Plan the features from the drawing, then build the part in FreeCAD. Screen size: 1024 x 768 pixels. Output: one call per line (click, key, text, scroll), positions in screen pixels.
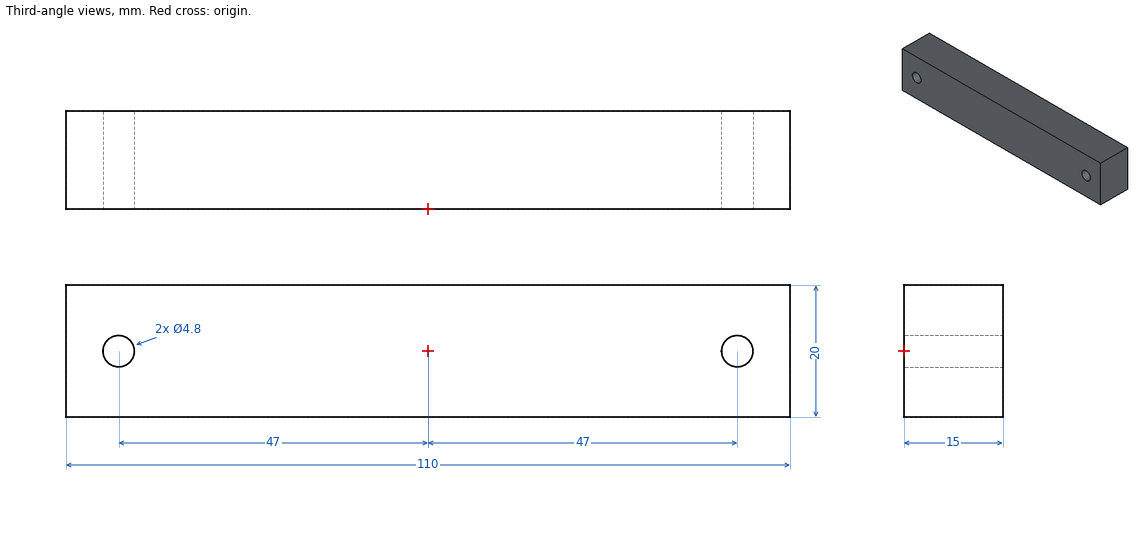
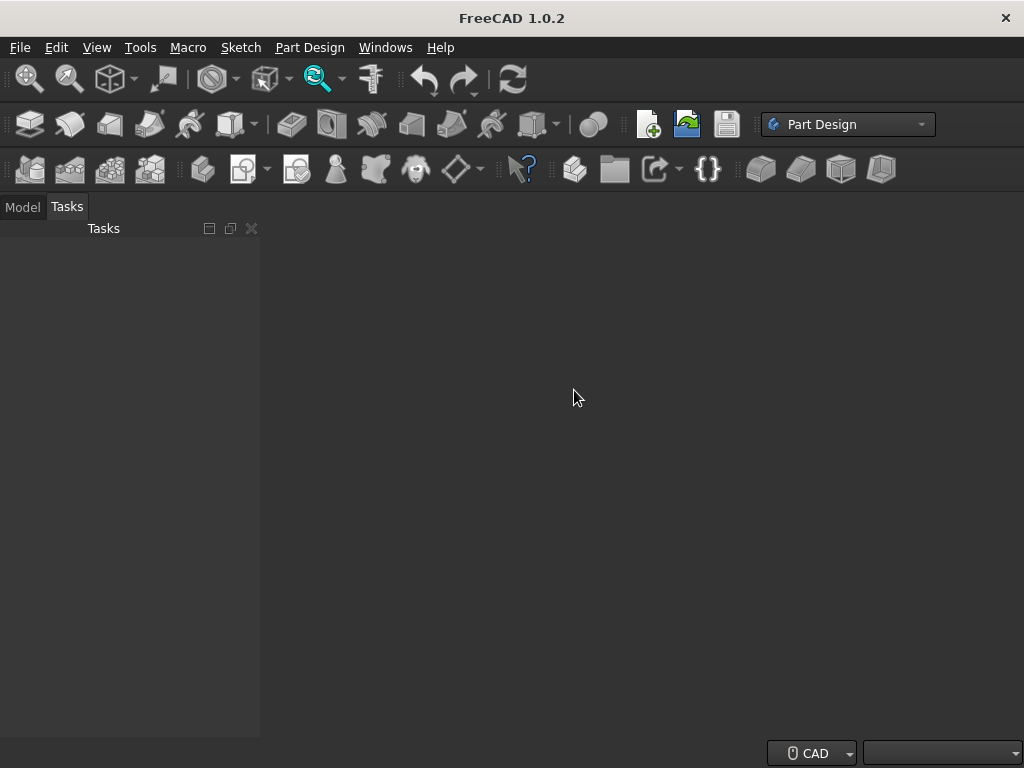
key(ctrl+n)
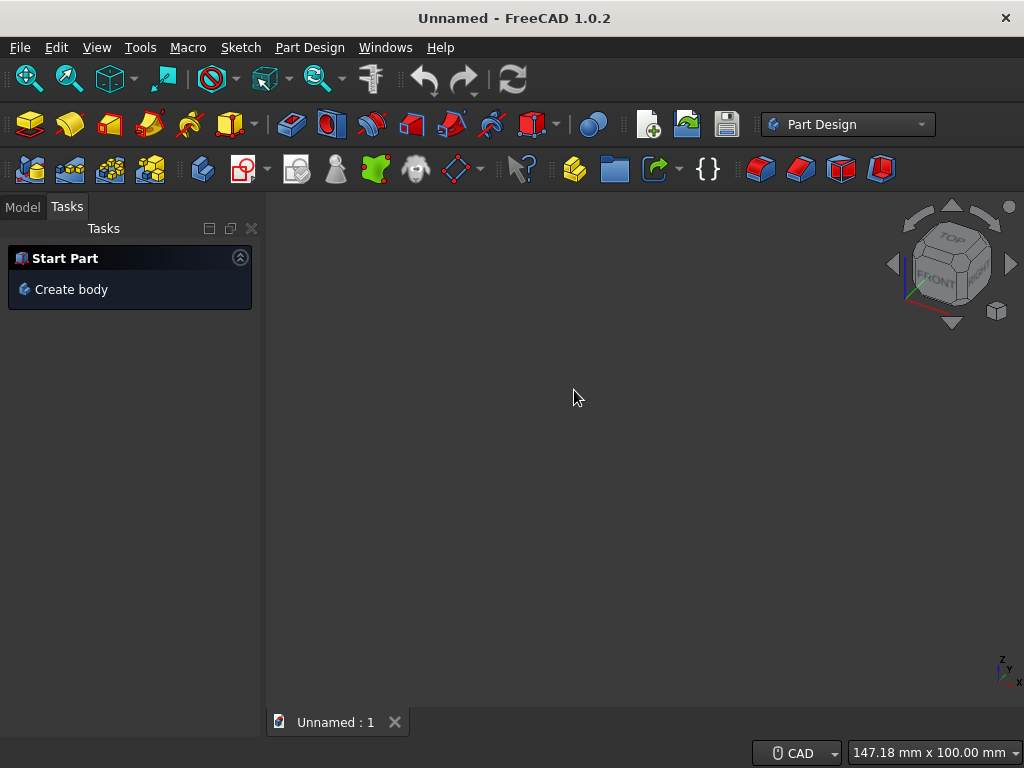
click(244, 170)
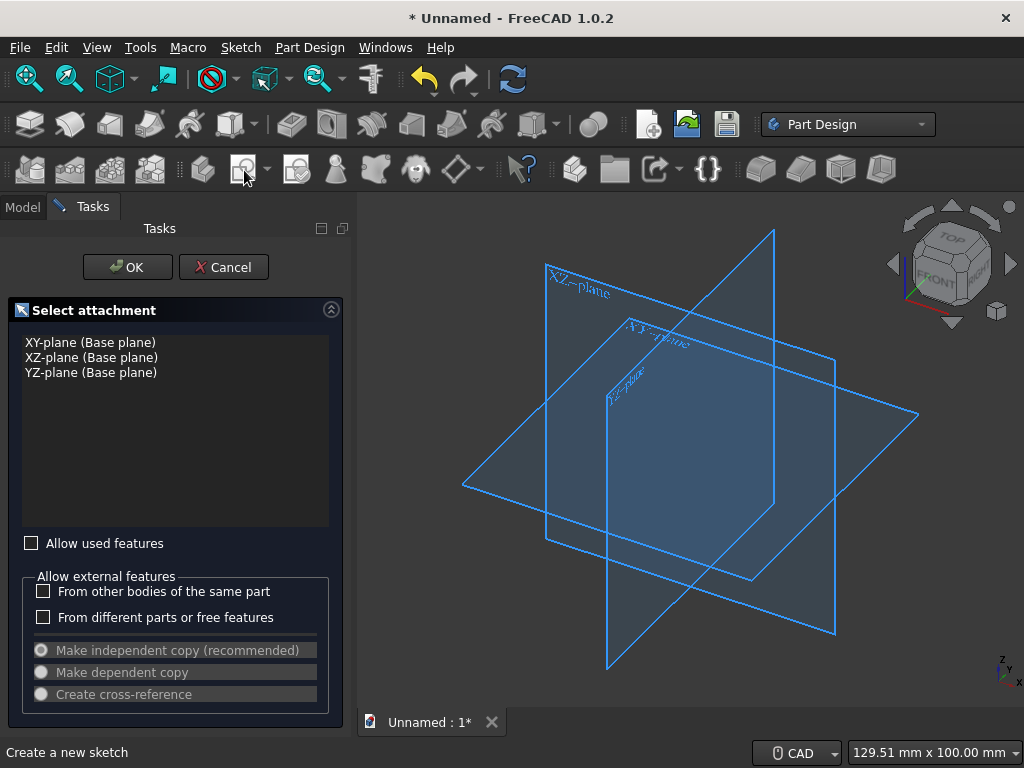
click(82, 358)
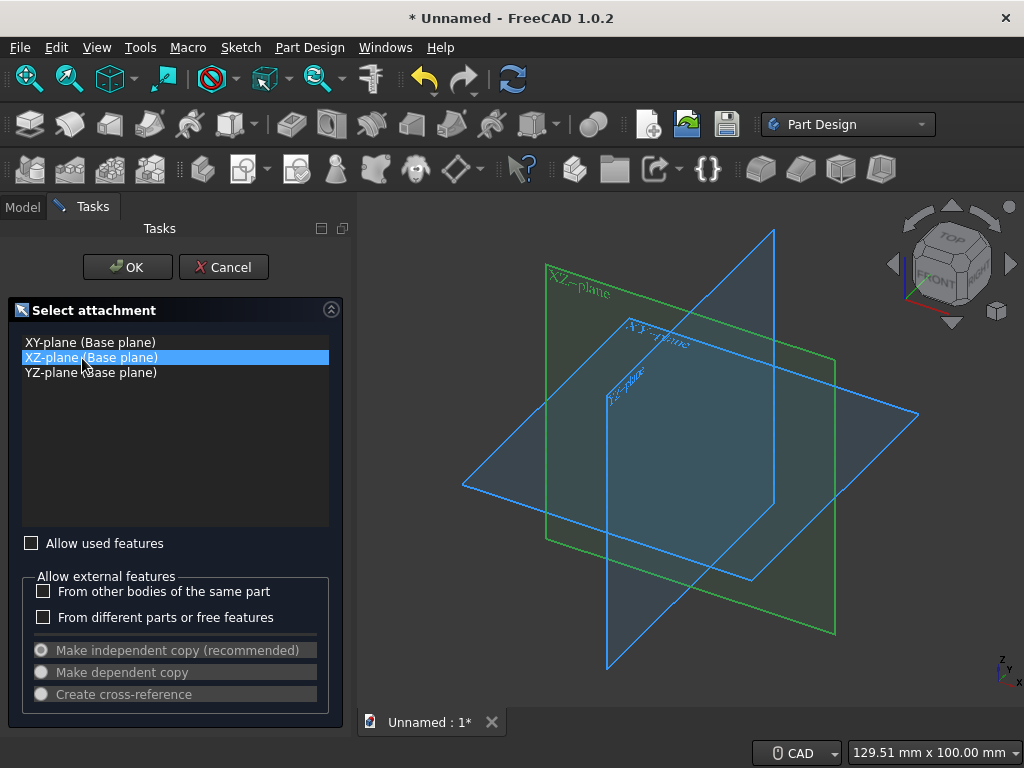
click(128, 267)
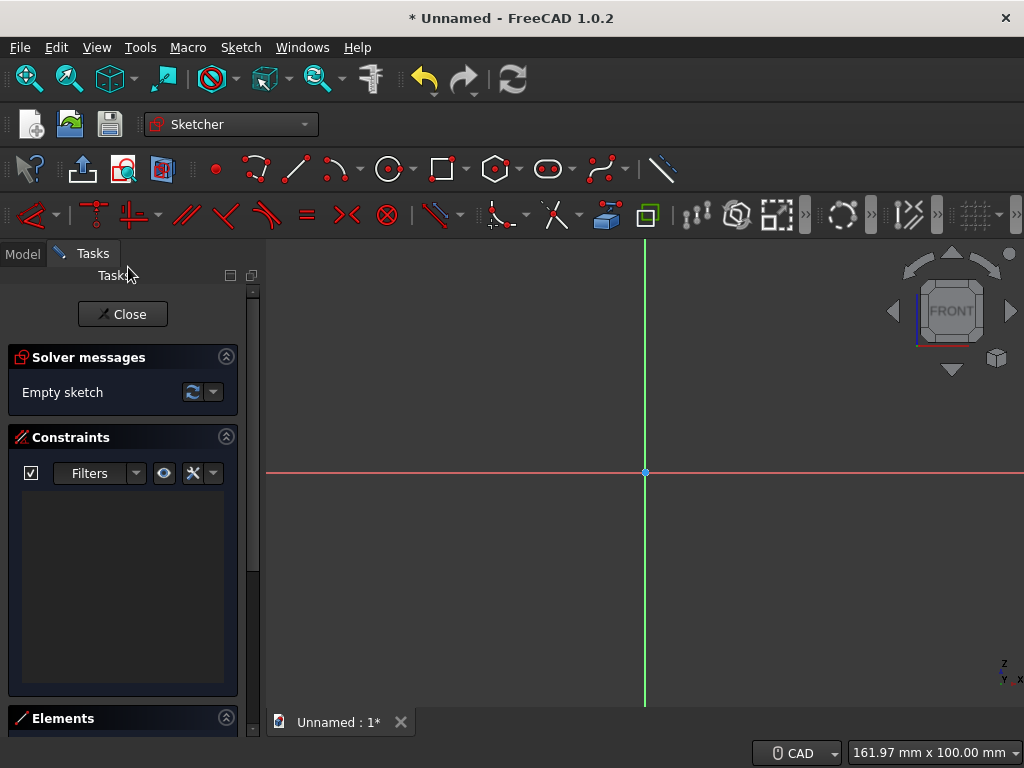
scroll(294, 473, down, 1)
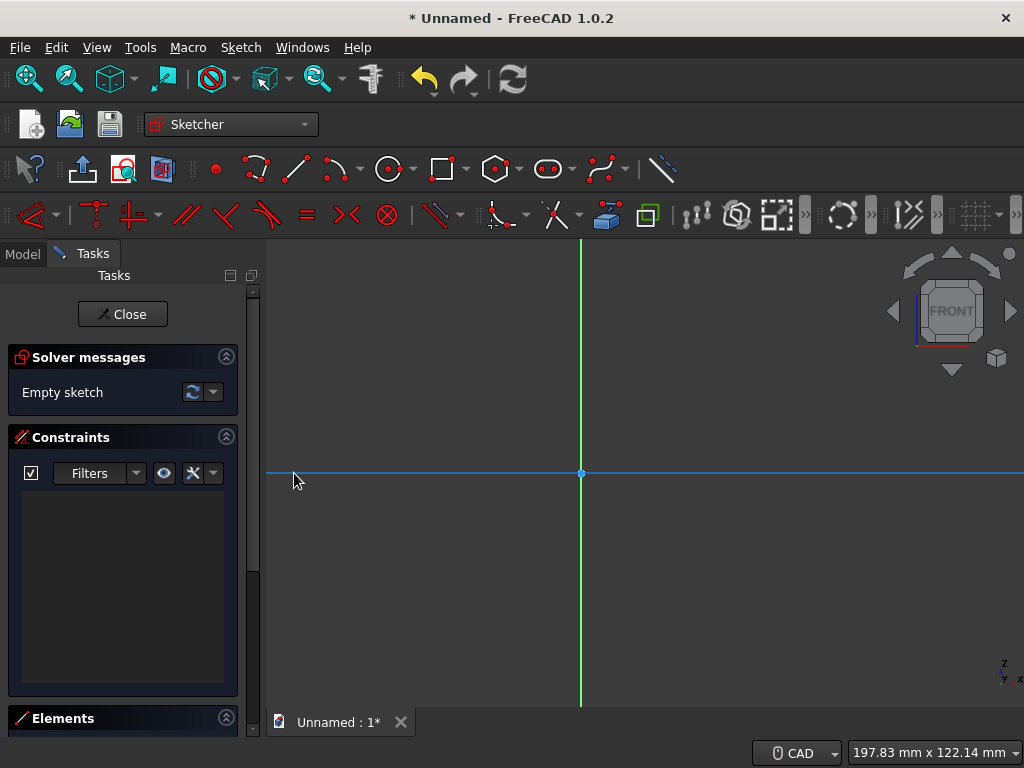
key(g)
key(v)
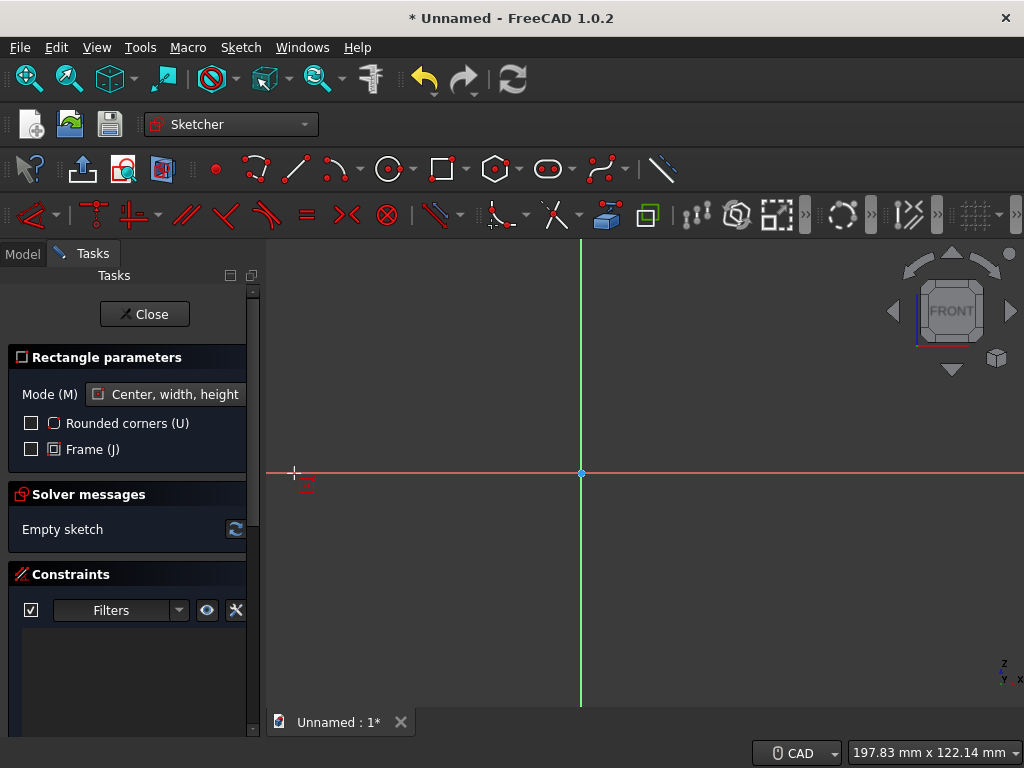
click(581, 473)
move(792, 435)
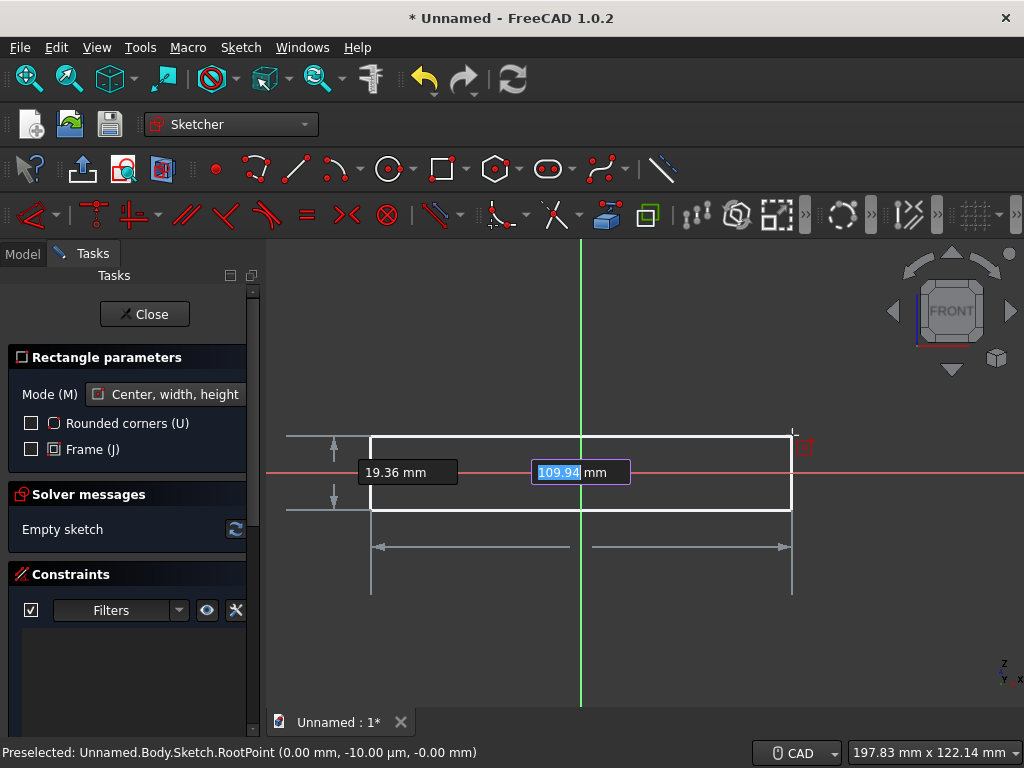
text(110)
key(Tab)
text(20)
key(Return)
key(Escape)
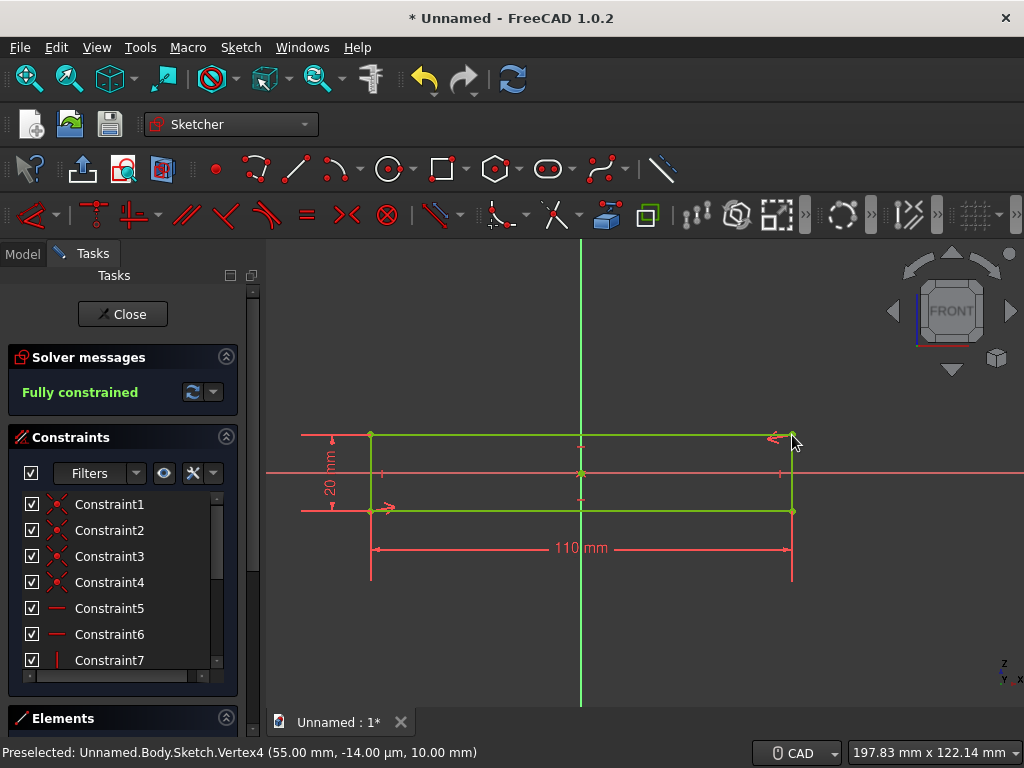
click(123, 314)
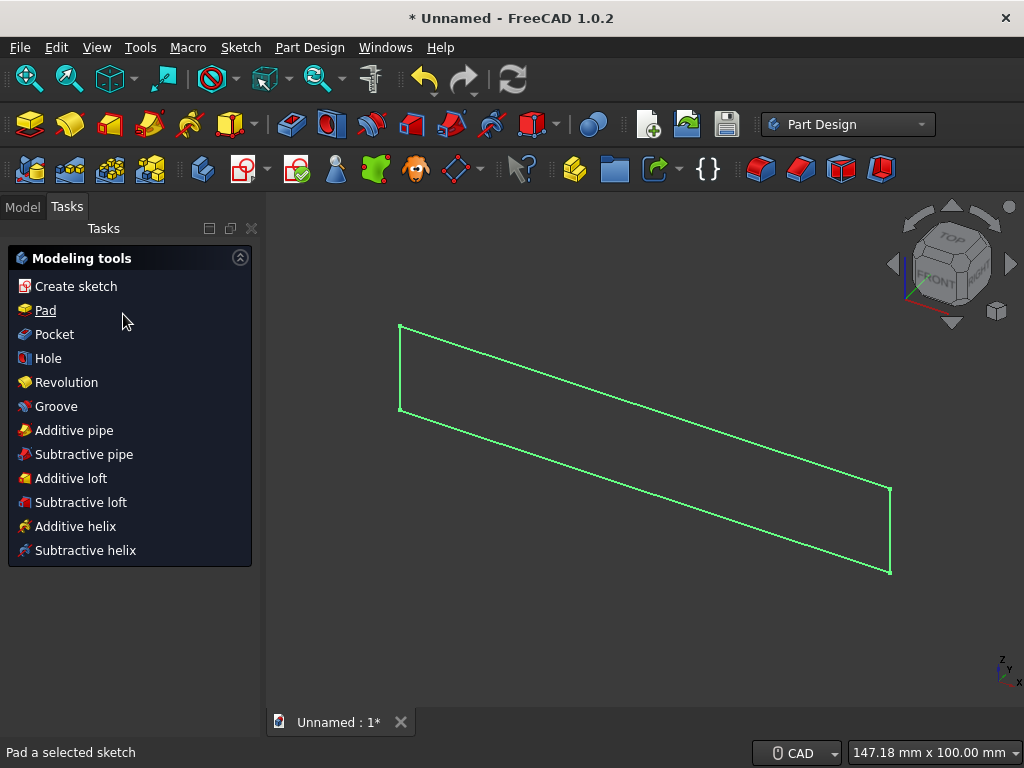
click(30, 124)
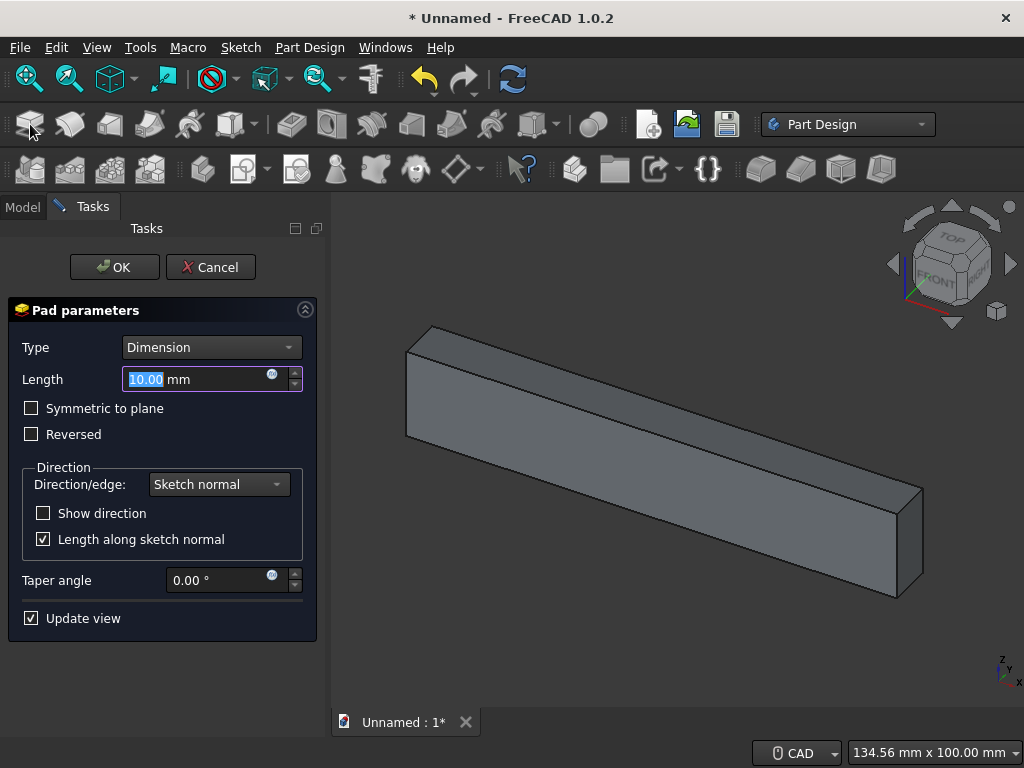
text(15)
key(Tab)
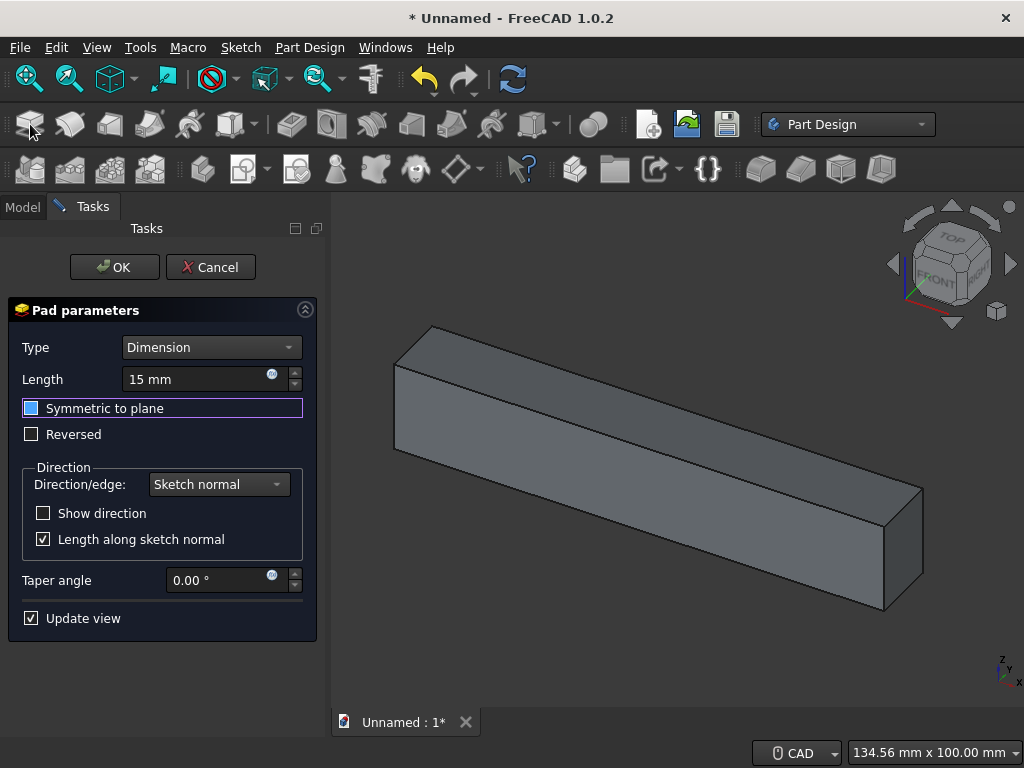
click(30, 434)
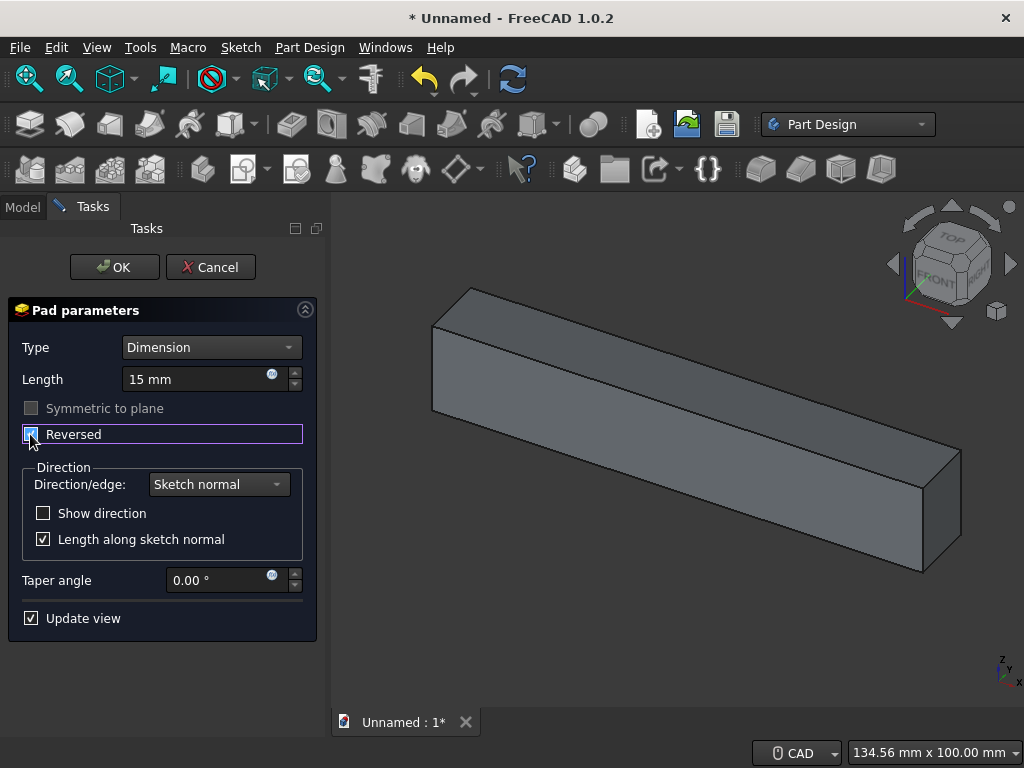
click(115, 267)